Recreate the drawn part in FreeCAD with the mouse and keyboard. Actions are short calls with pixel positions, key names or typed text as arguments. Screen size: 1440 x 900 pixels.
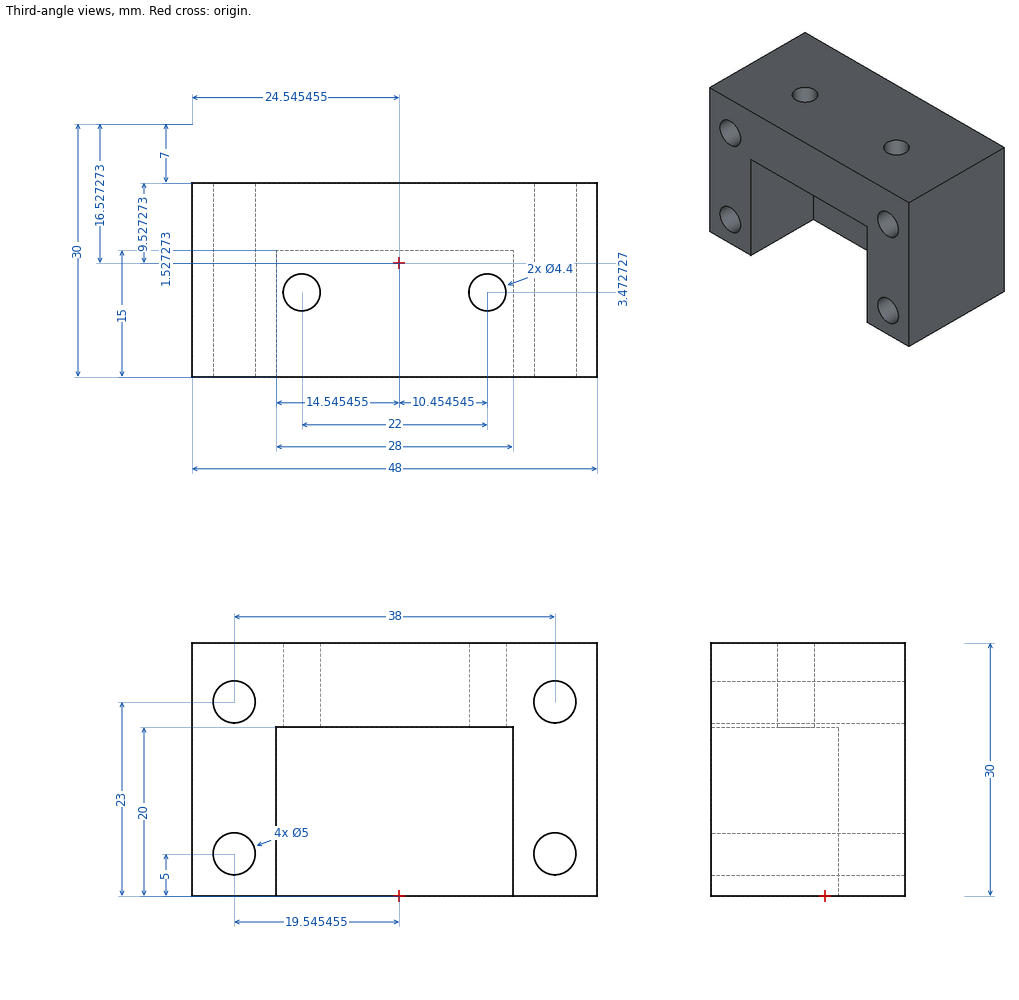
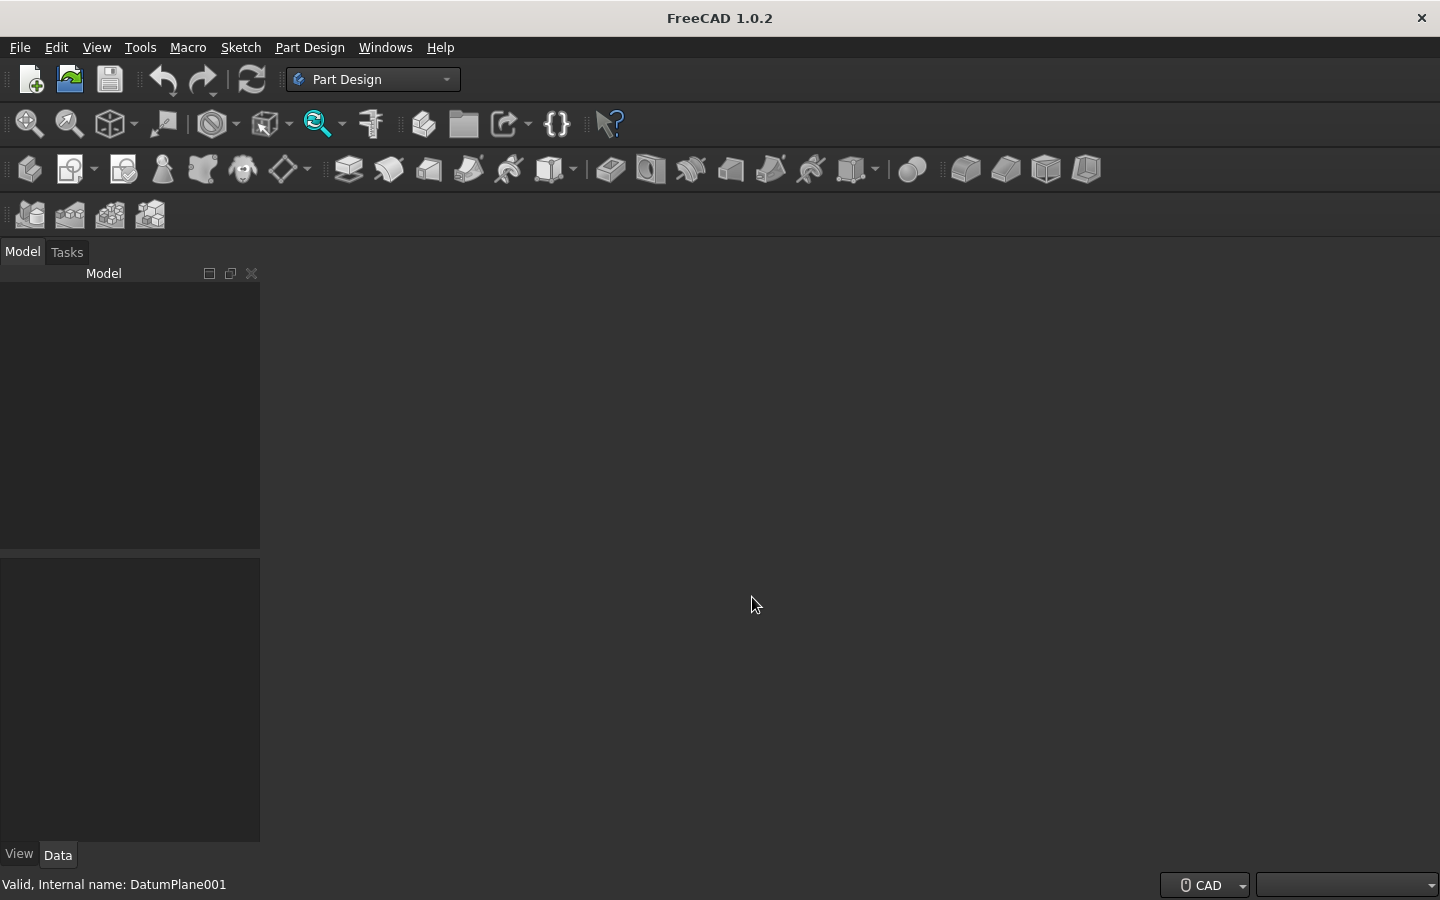
click(30, 80)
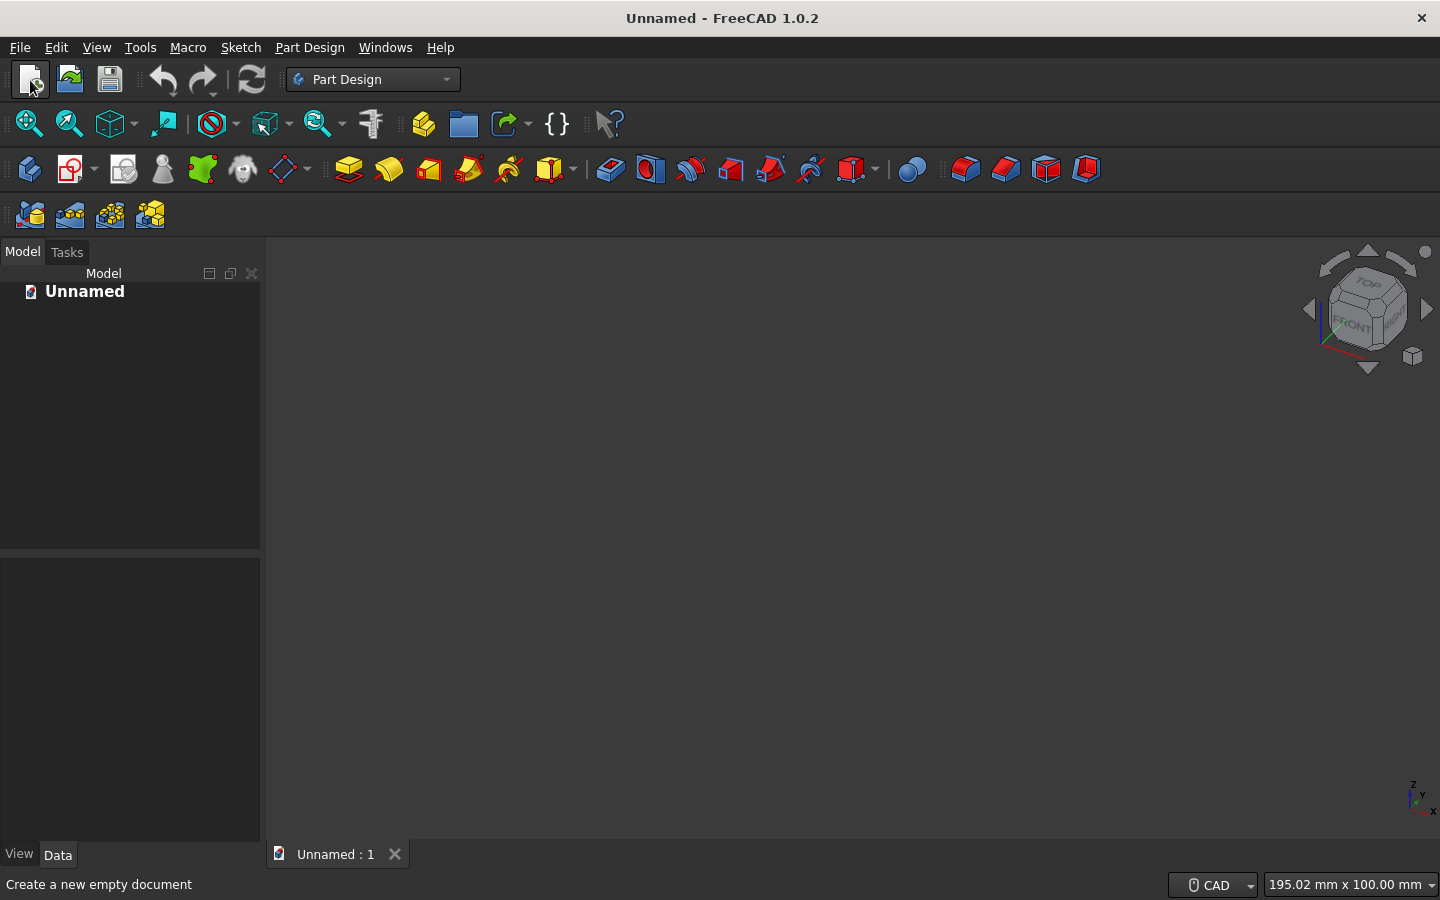
click(70, 170)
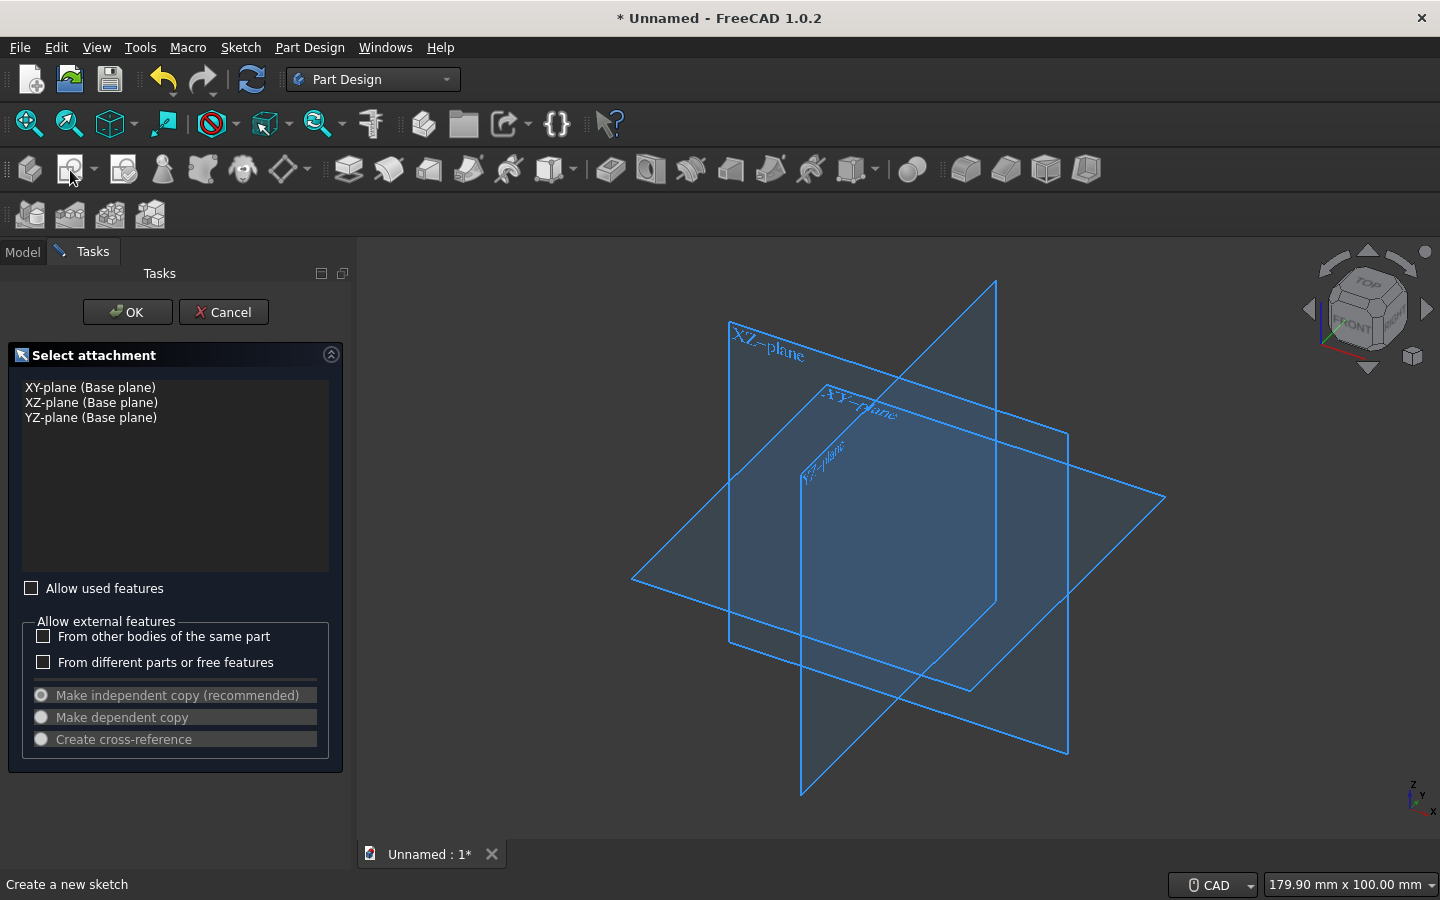
click(82, 388)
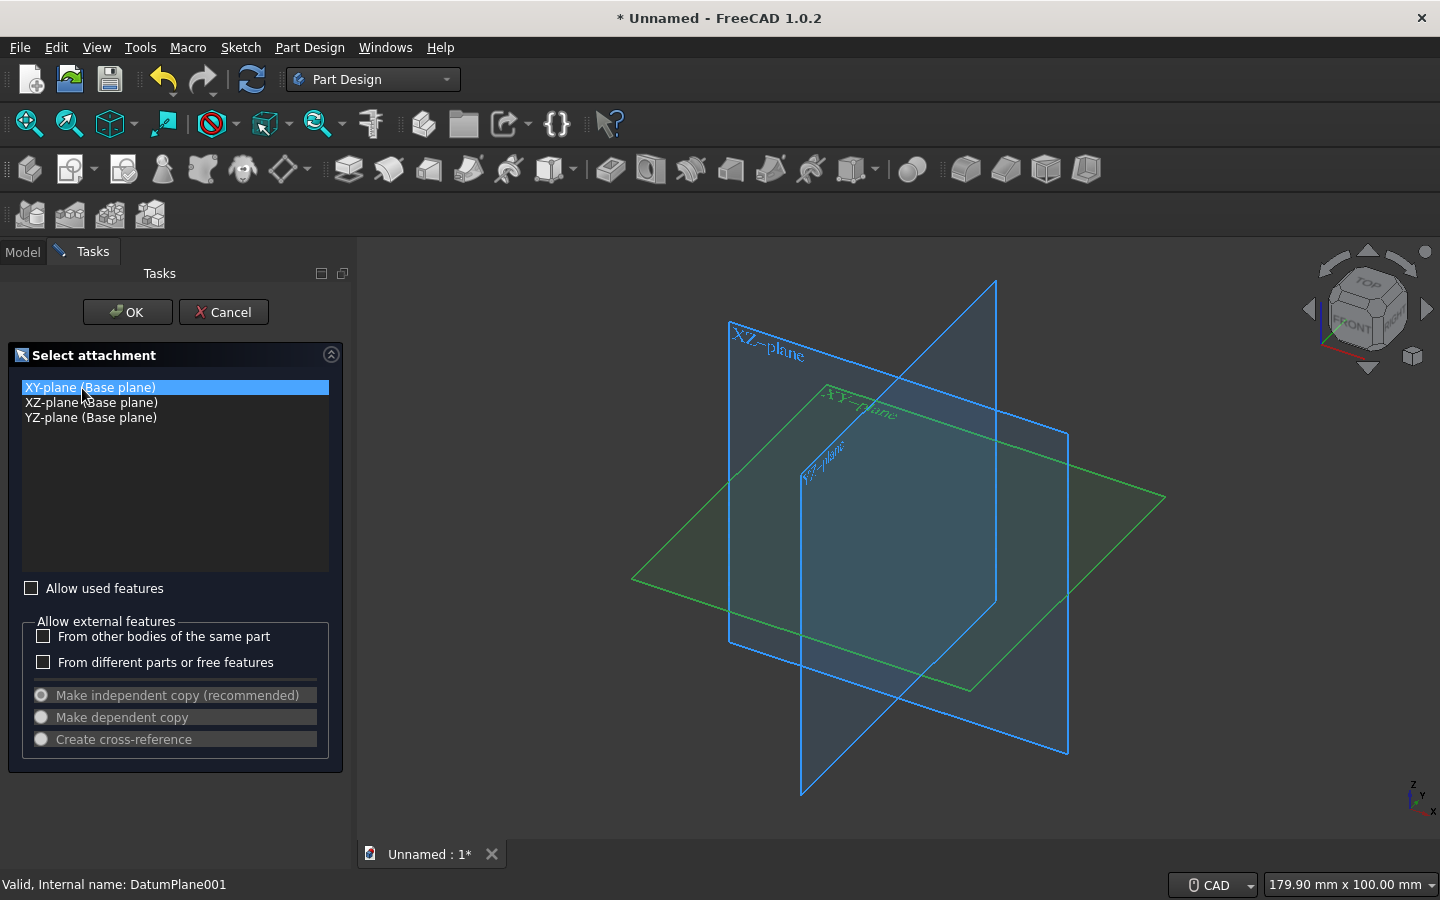
click(128, 312)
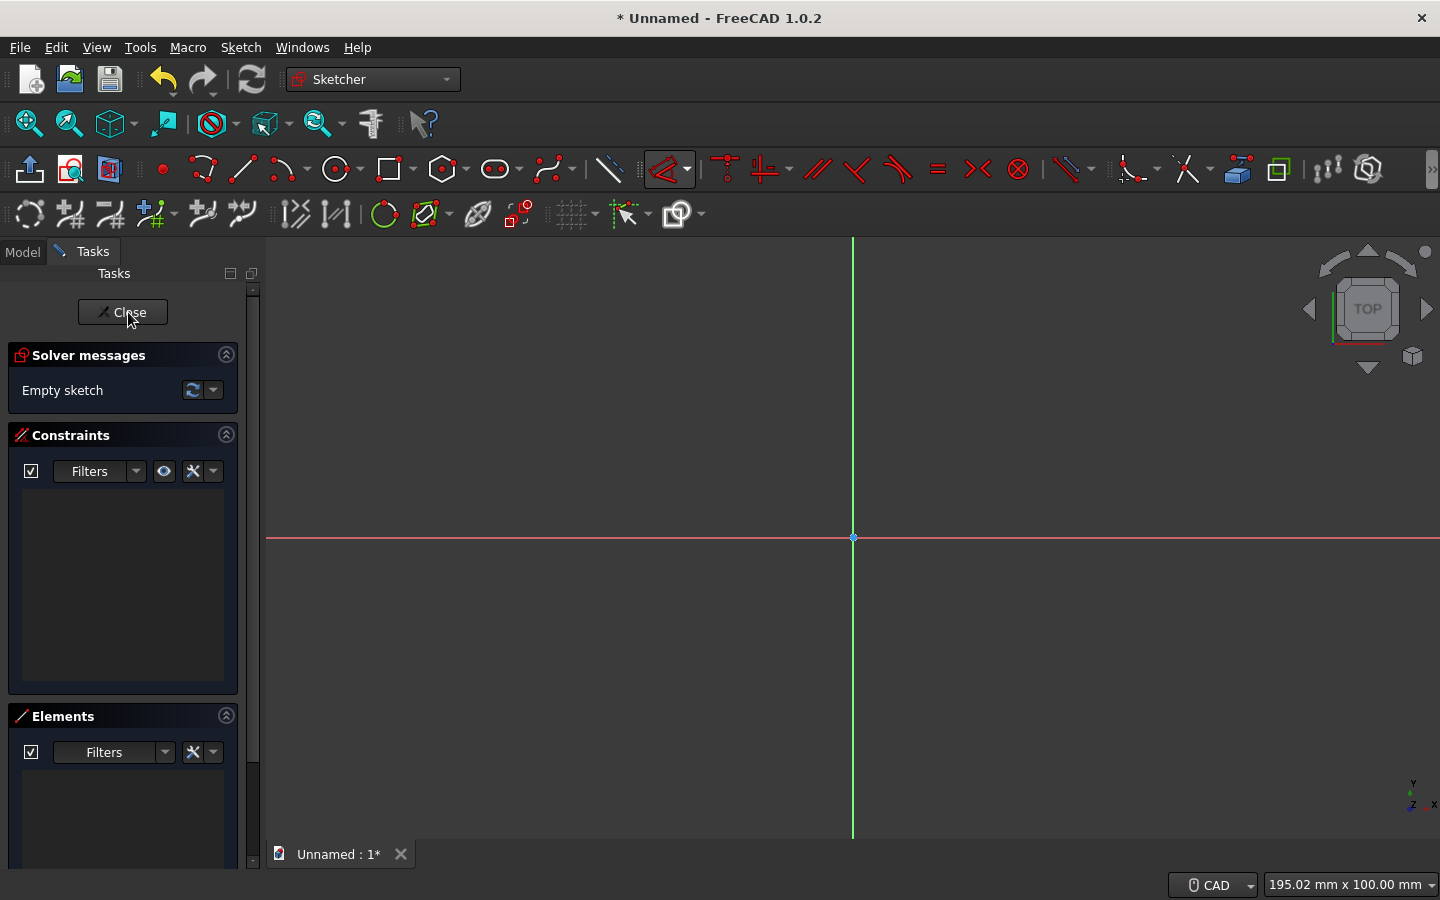
scroll(903, 521, up, 4)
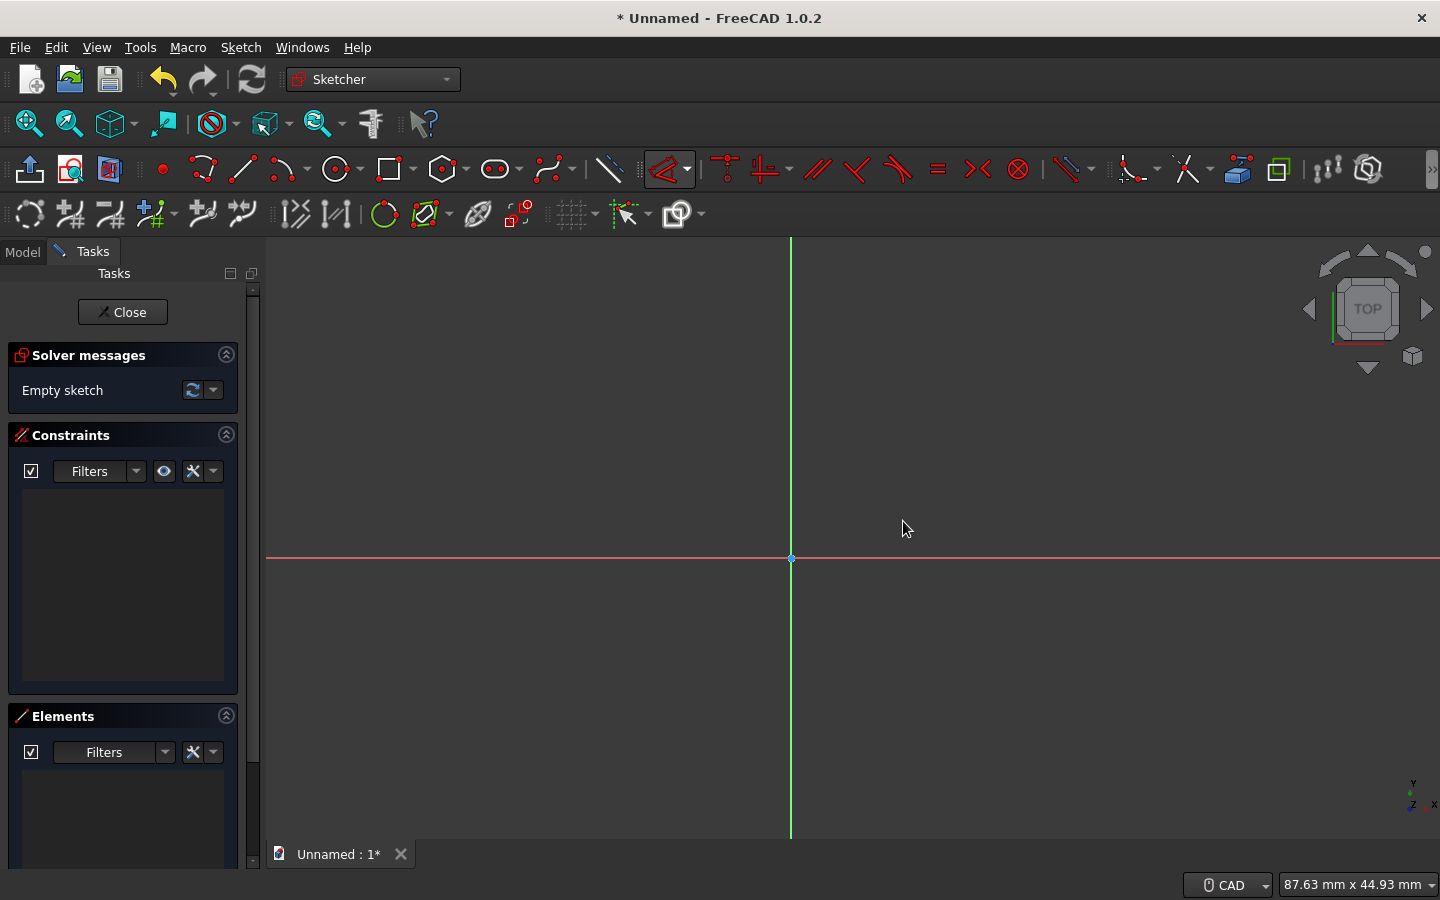
click(390, 170)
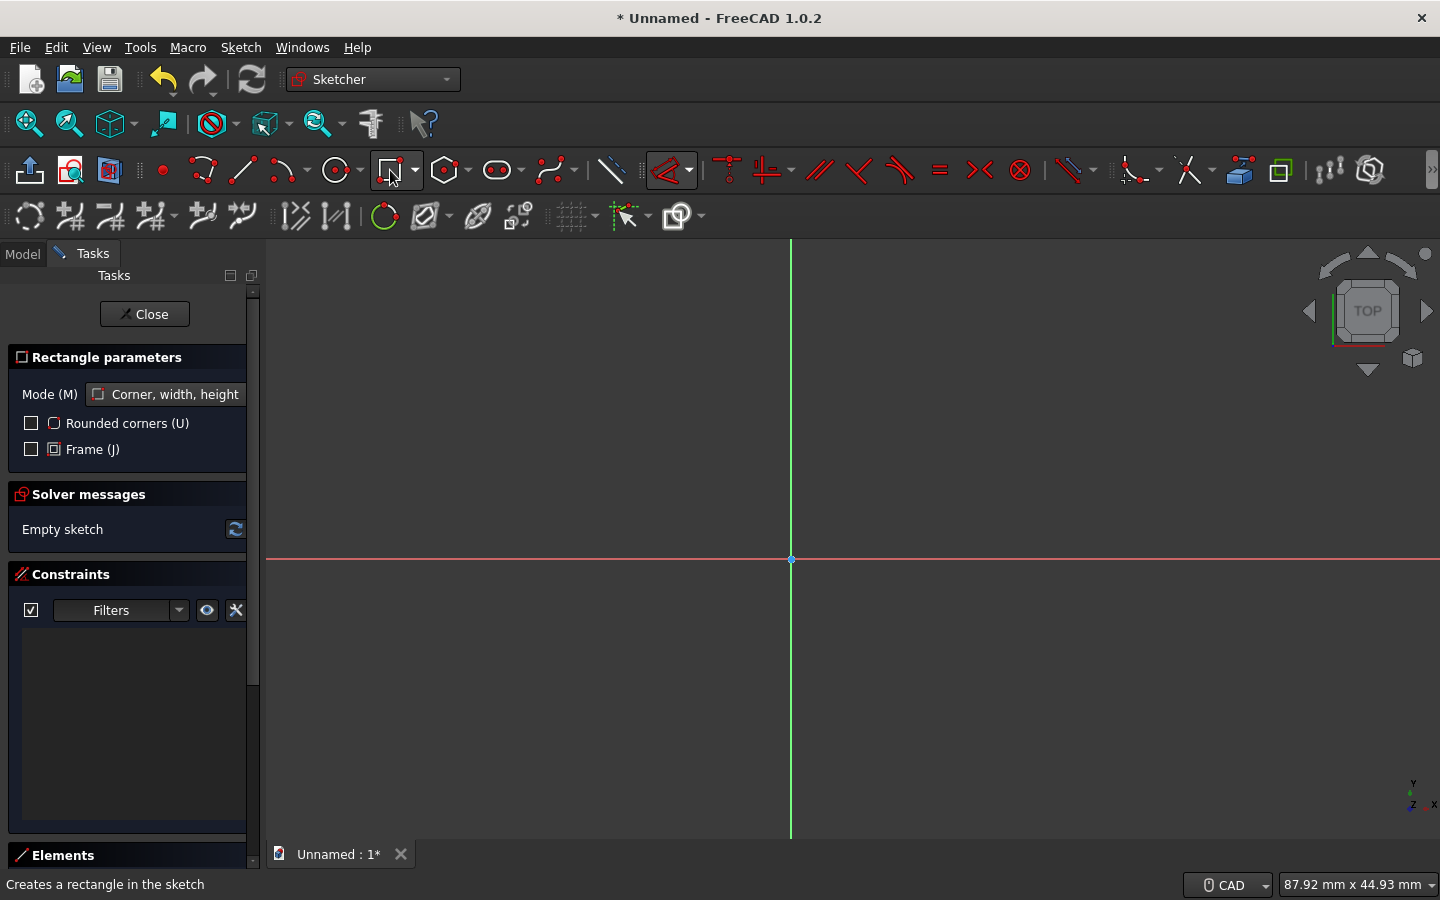
click(464, 338)
click(1104, 739)
key(Escape)